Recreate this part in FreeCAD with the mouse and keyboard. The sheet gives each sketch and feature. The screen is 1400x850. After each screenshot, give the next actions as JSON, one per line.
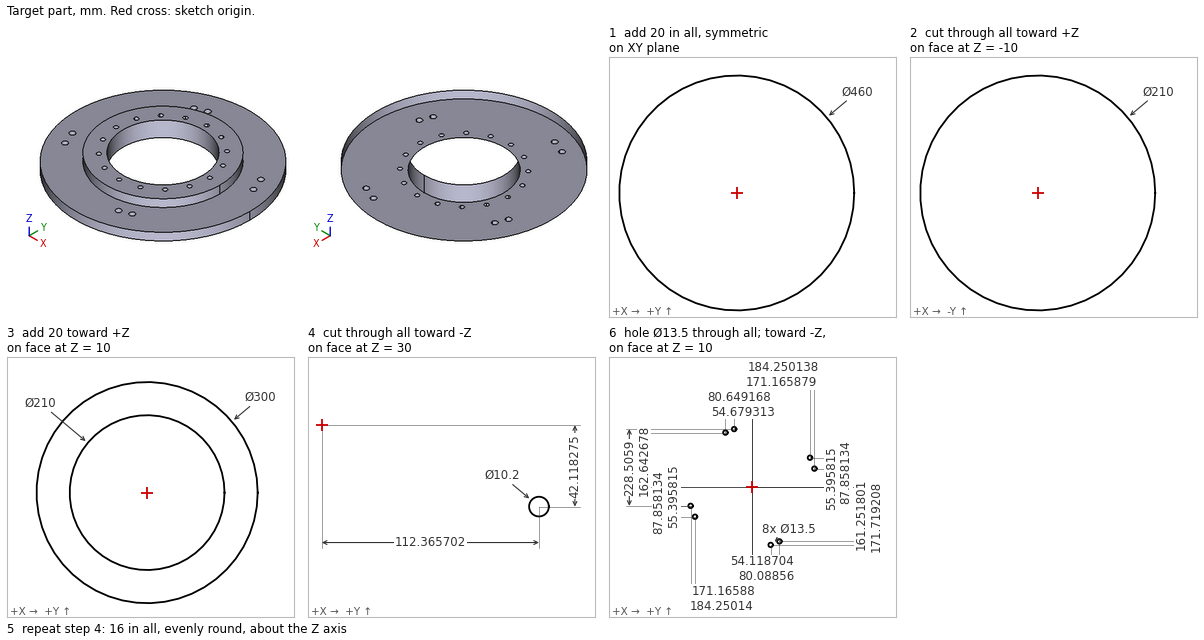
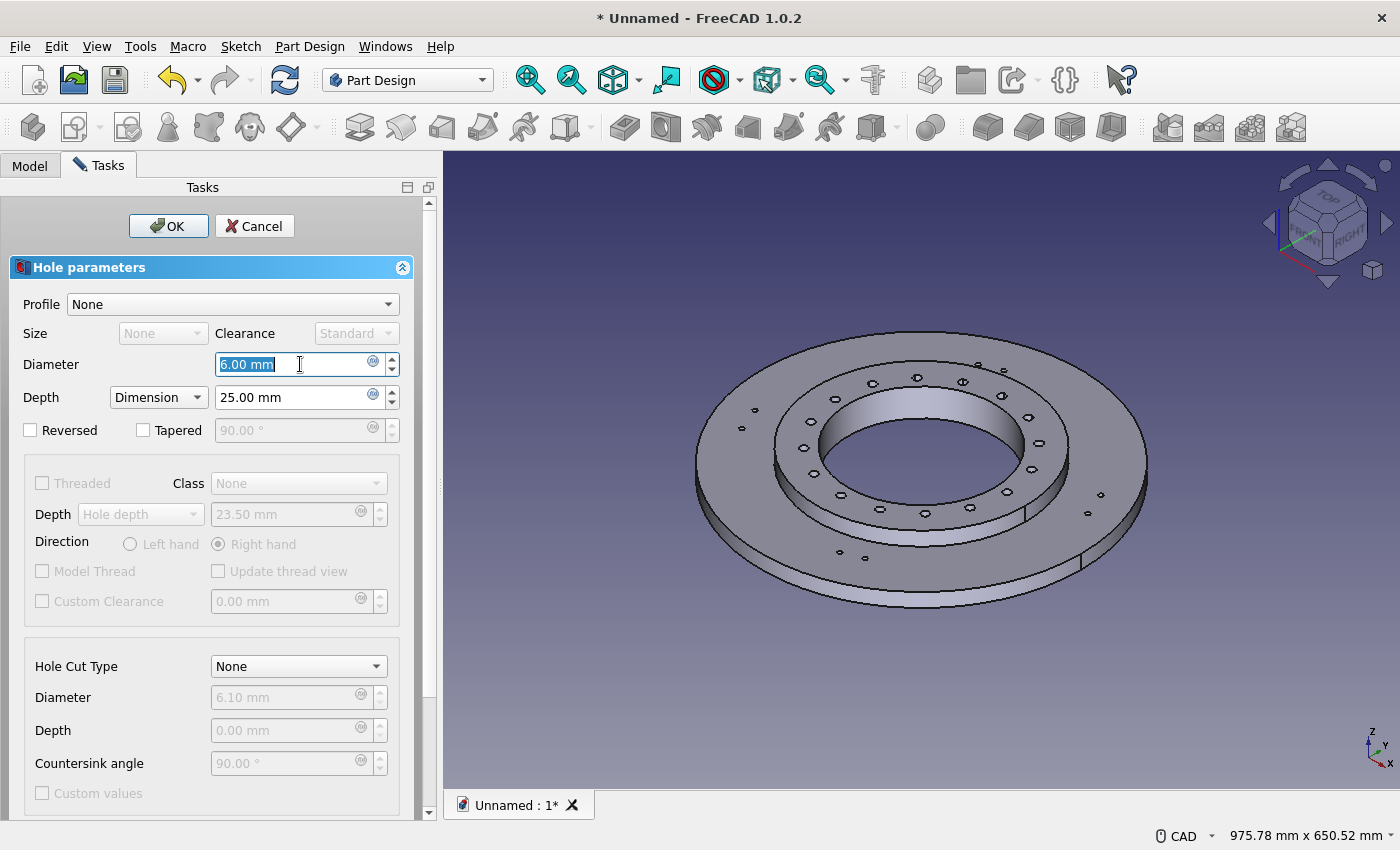
{"action": "type", "text": "13.5"}
{"action": "key", "text": "Tab"}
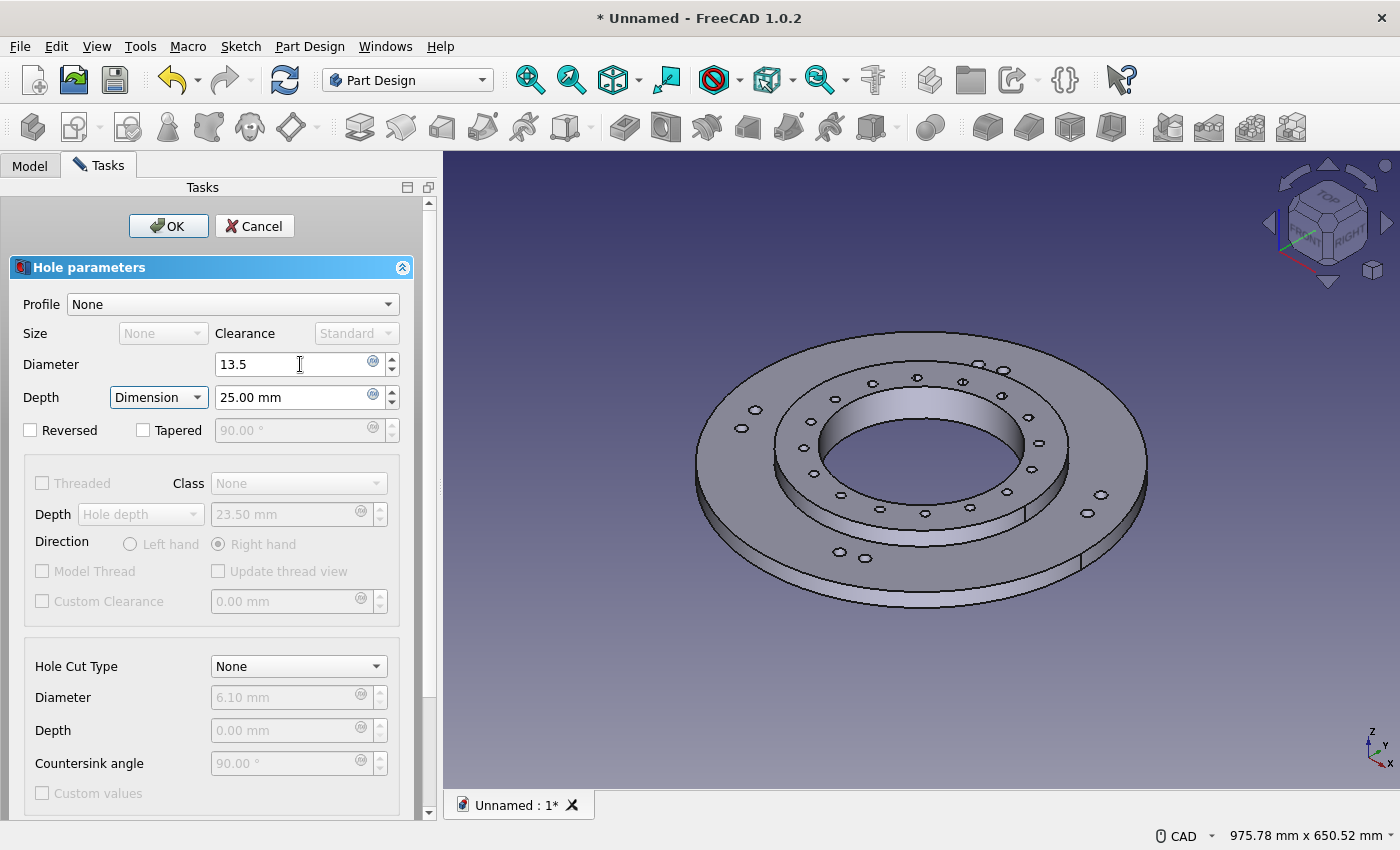
{"action": "left_click", "coordinate": [160, 398]}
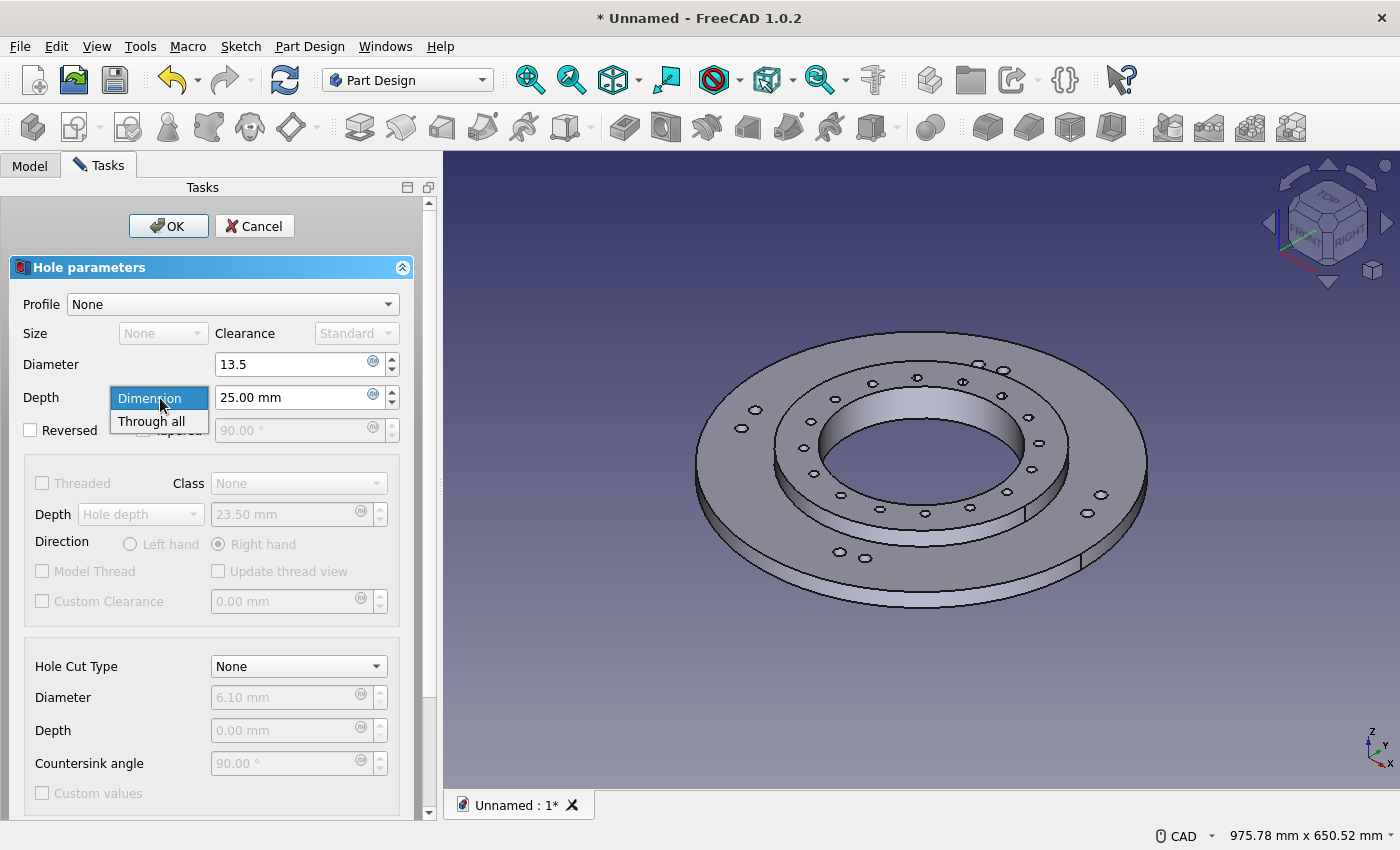
{"action": "left_click", "coordinate": [158, 422]}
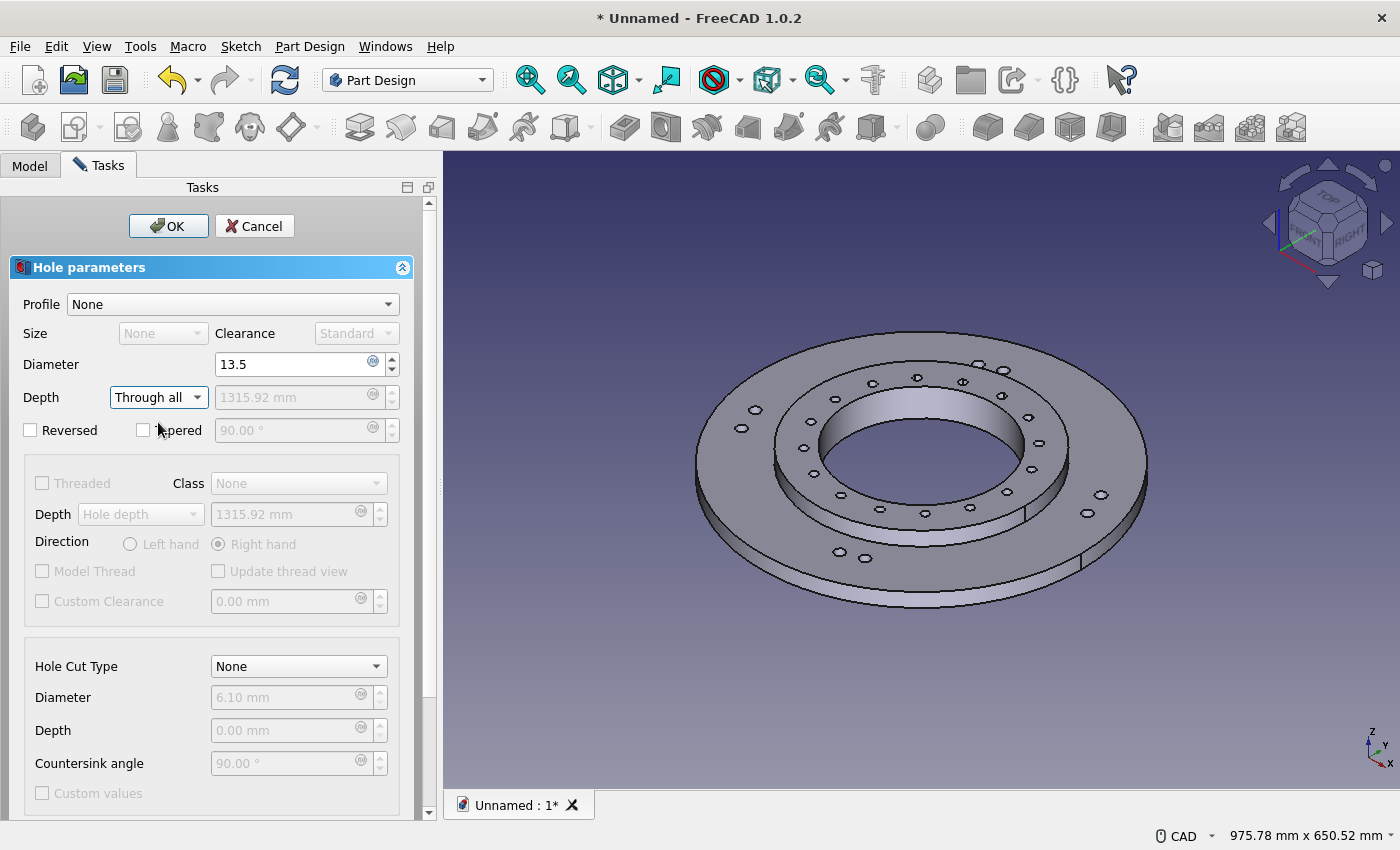
{"action": "left_click", "coordinate": [169, 226]}